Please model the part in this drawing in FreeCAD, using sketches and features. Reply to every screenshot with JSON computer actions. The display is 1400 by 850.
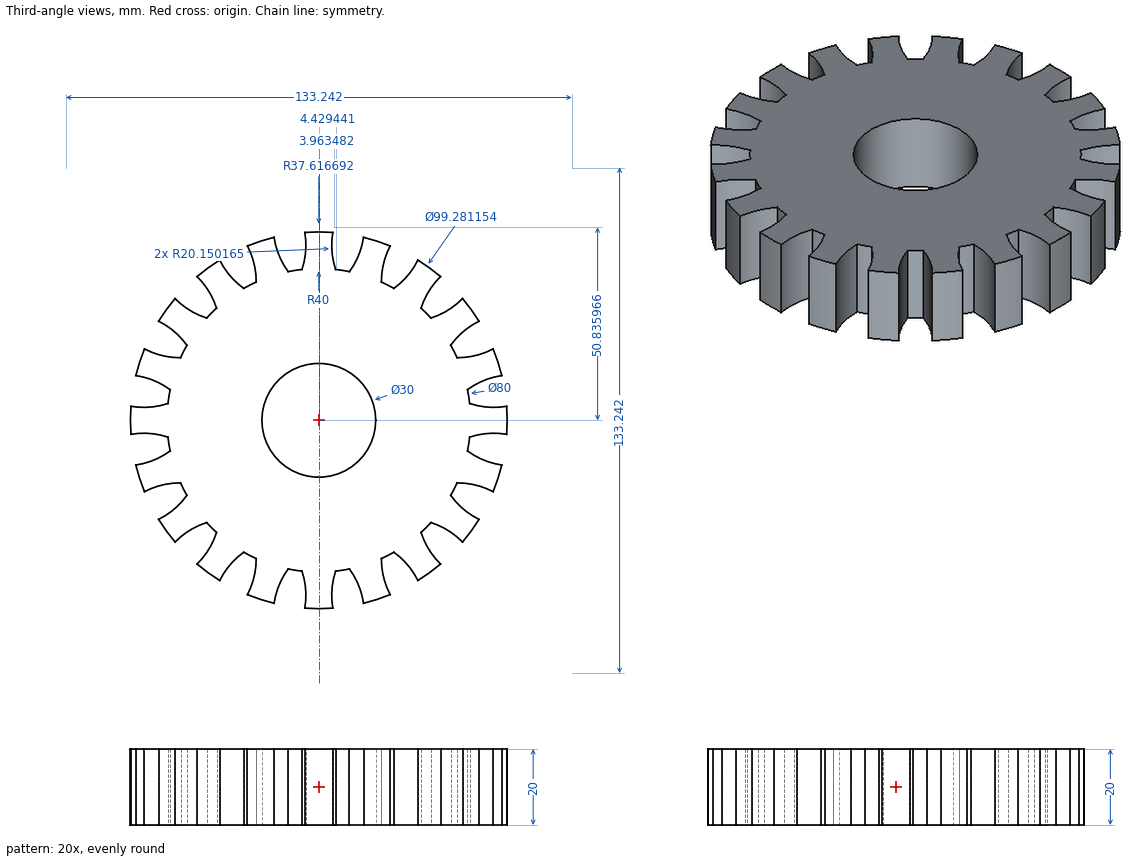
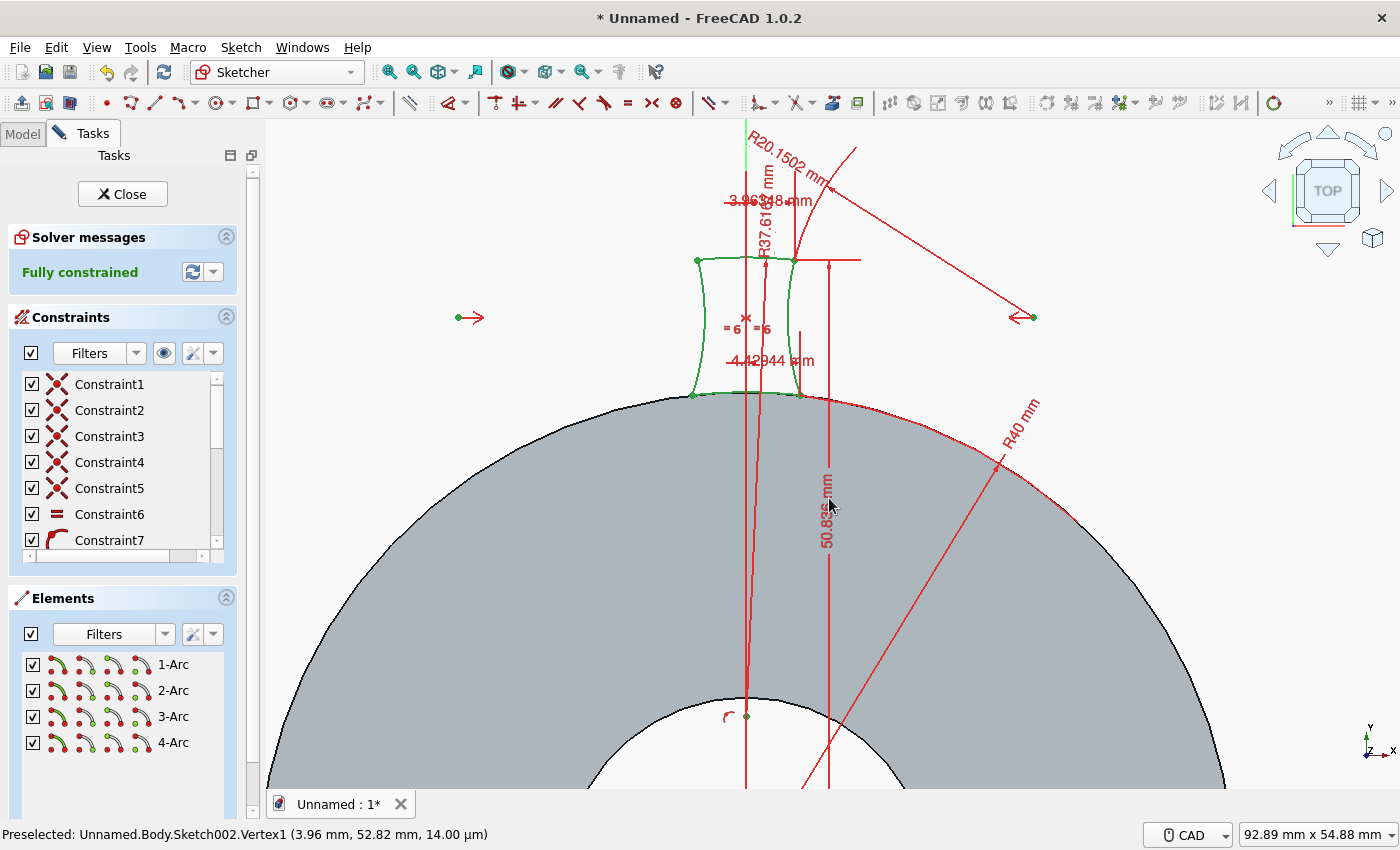
{"action": "left_click", "coordinate": [123, 194]}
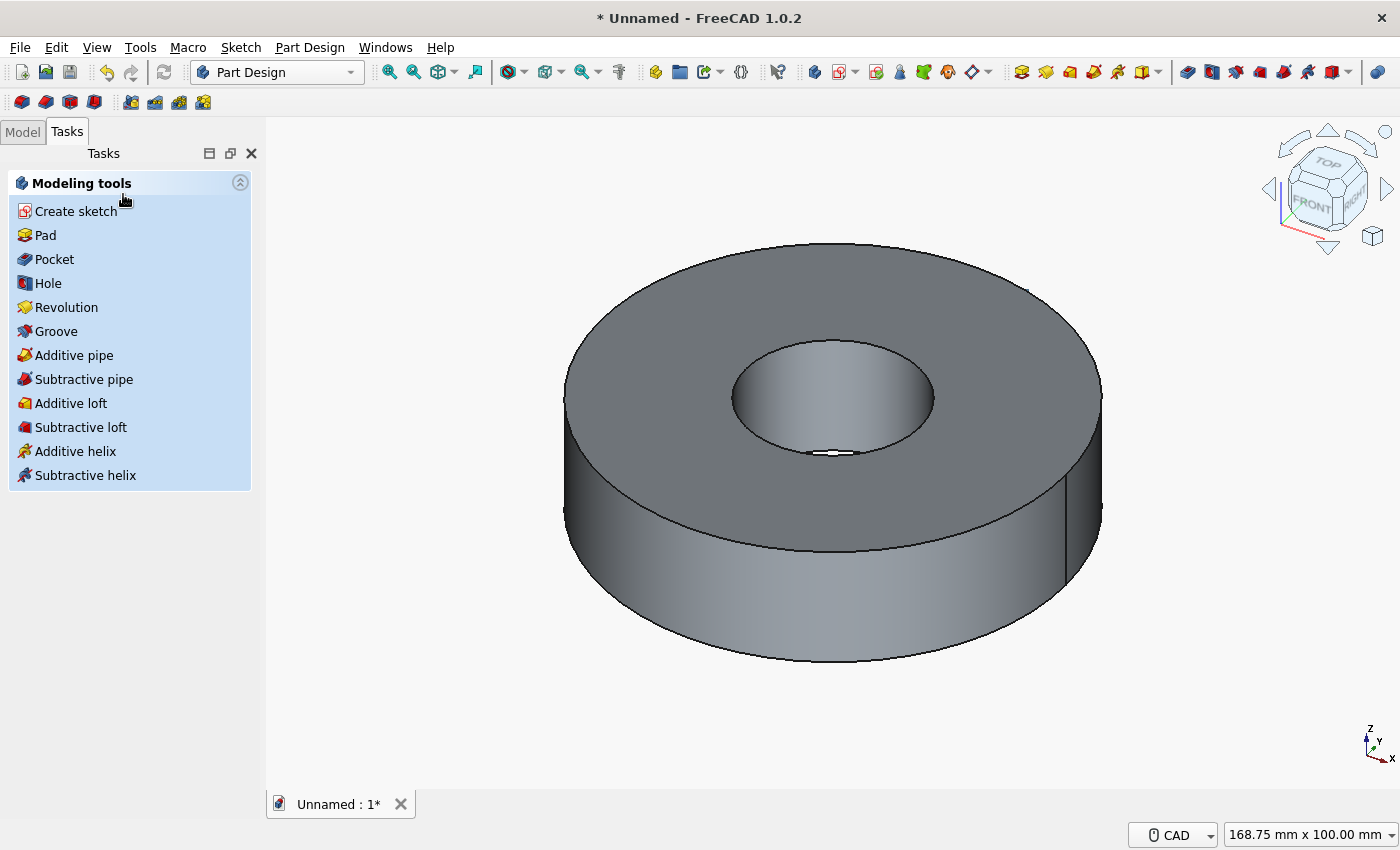
{"action": "left_click", "coordinate": [1022, 72]}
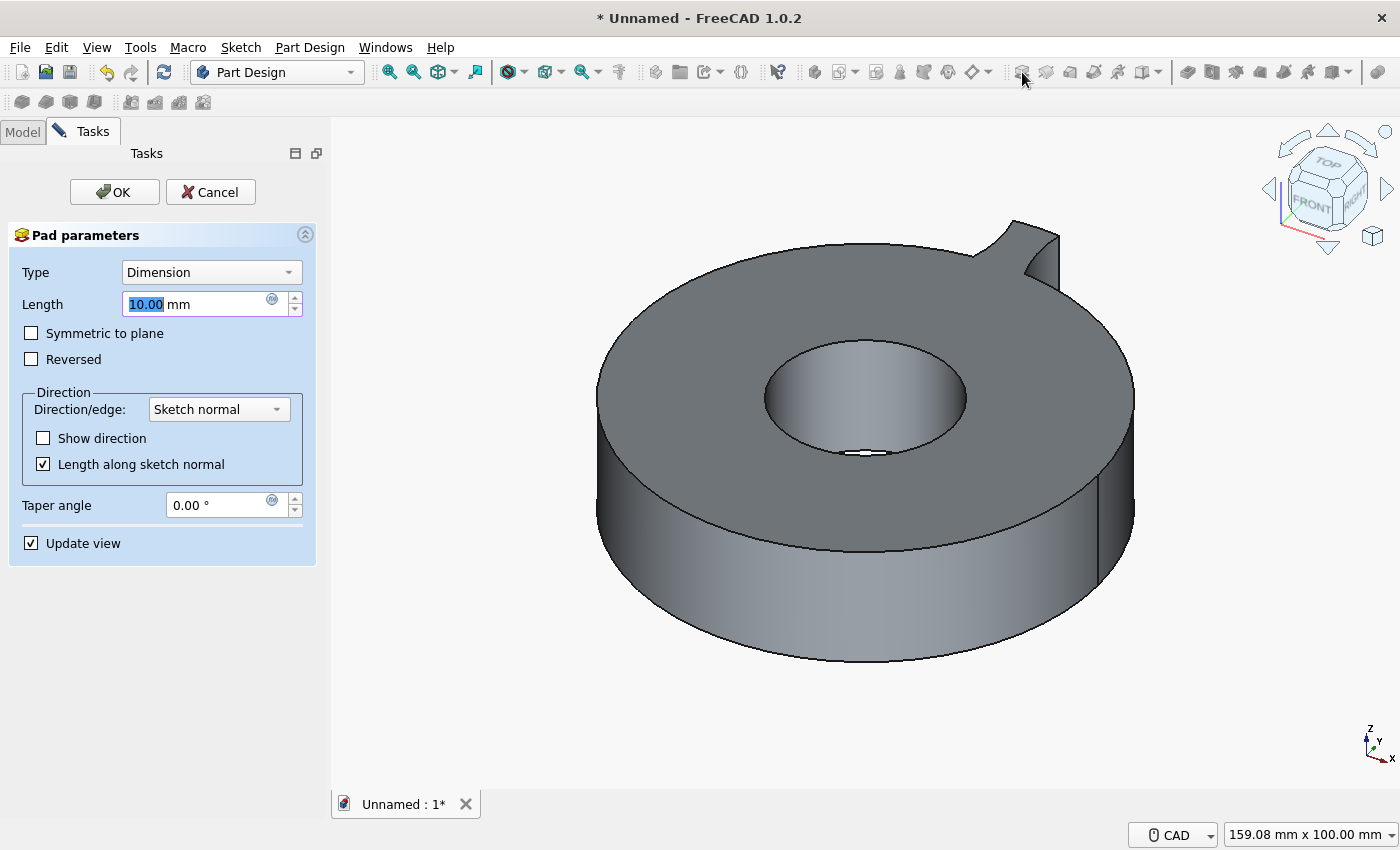
{"action": "type", "text": "20"}
{"action": "key", "text": "Tab"}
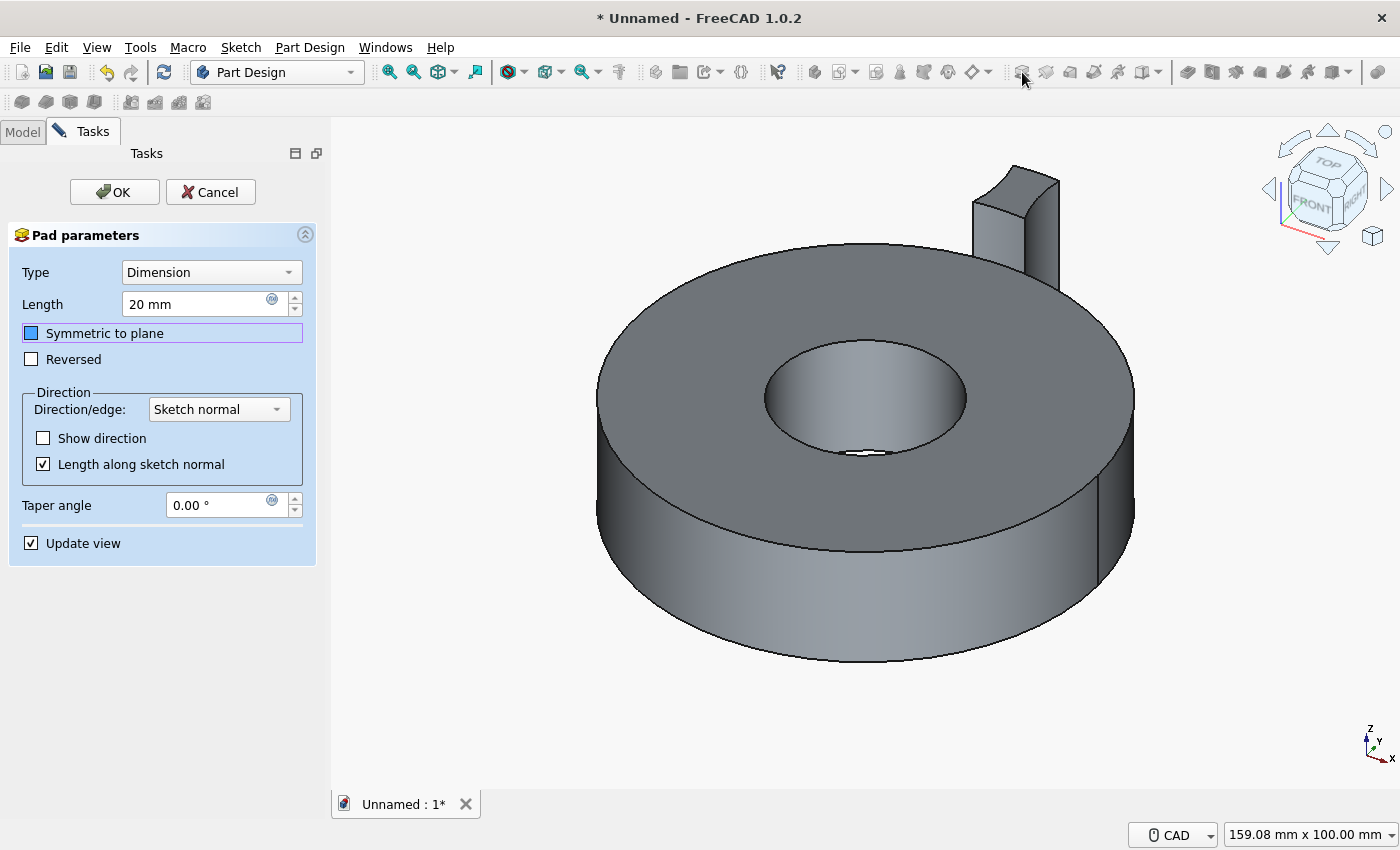
{"action": "left_click", "coordinate": [30, 333]}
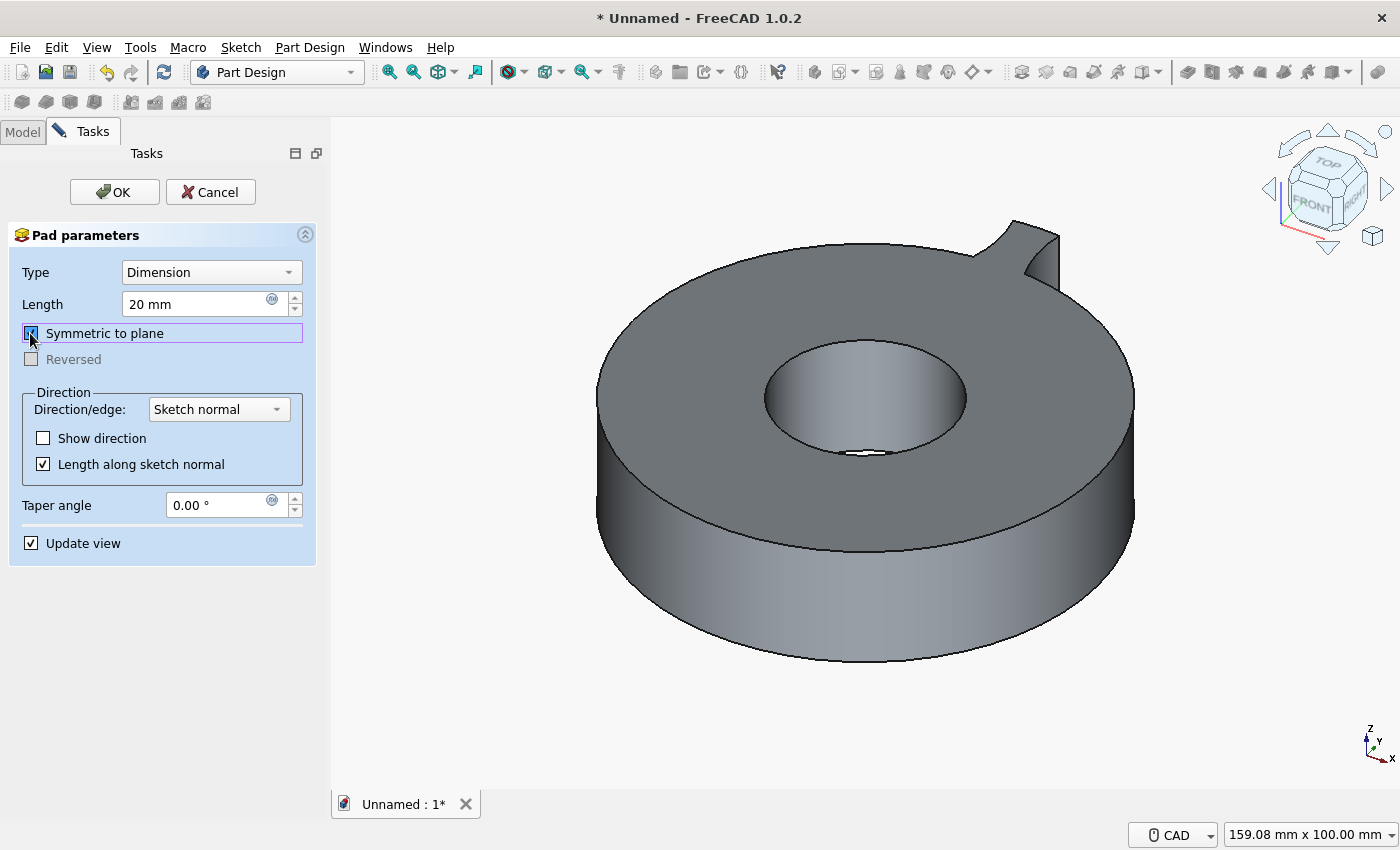
{"action": "left_click", "coordinate": [115, 192]}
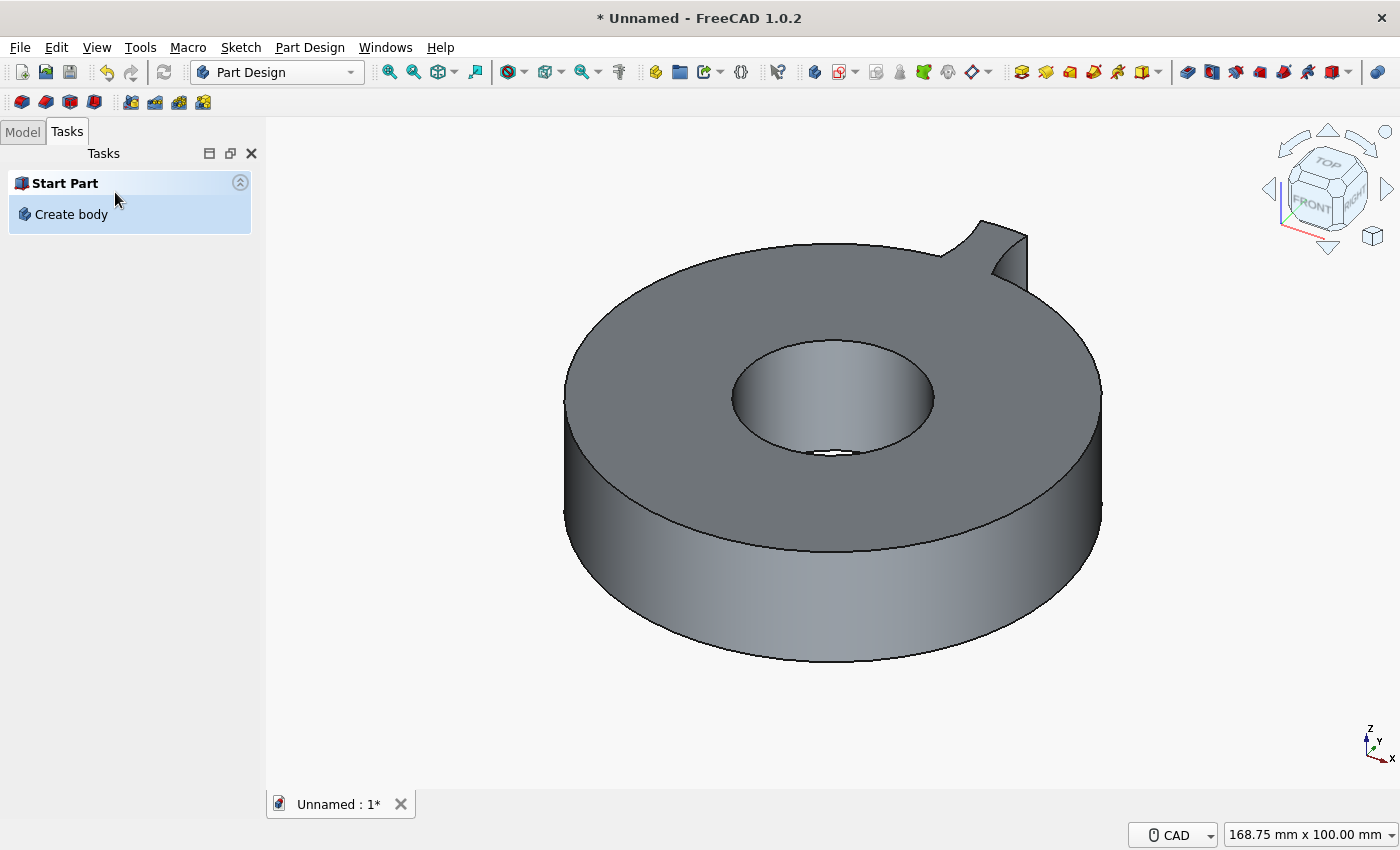
{"action": "left_click", "coordinate": [23, 131]}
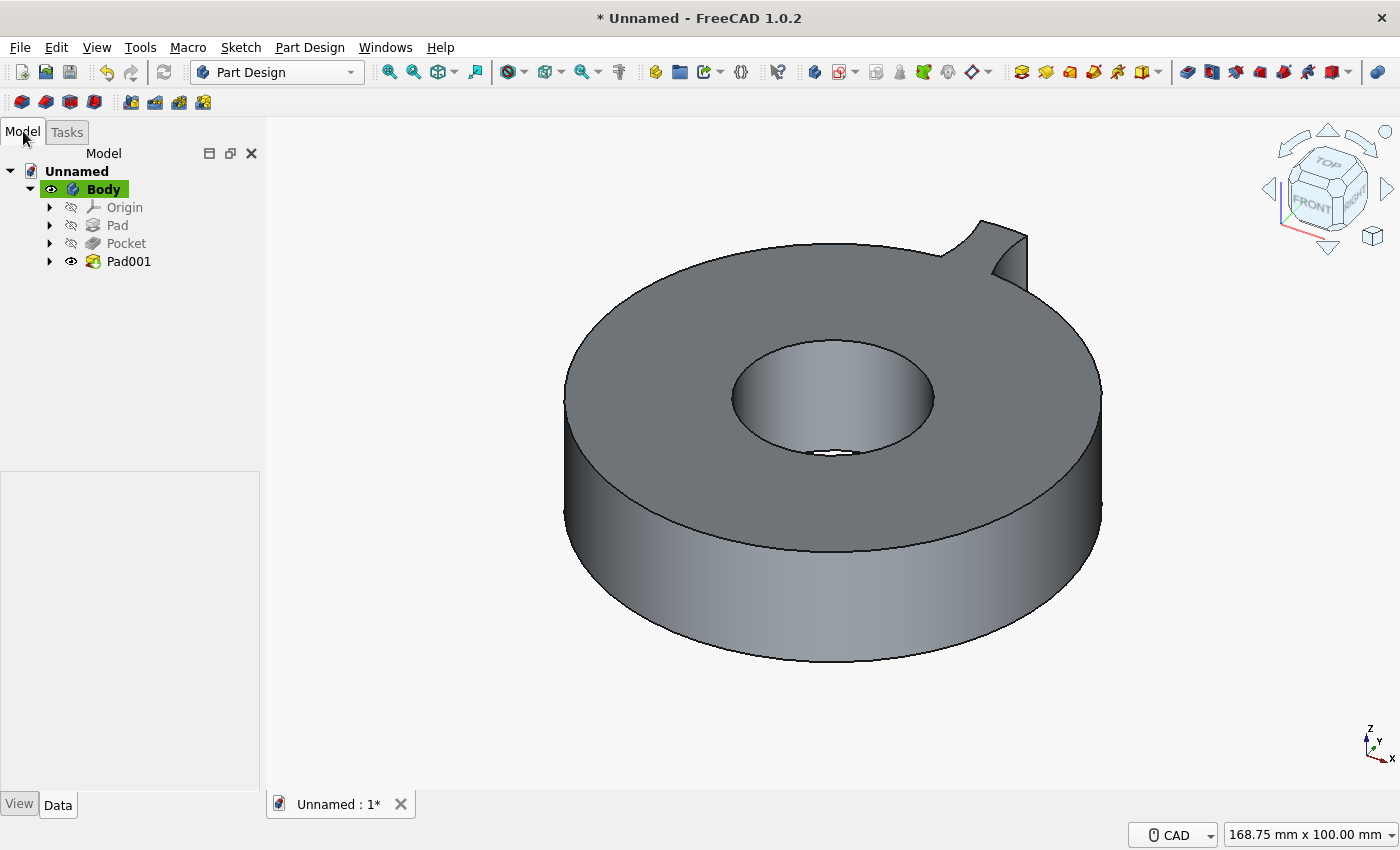
{"action": "left_click", "coordinate": [116, 261]}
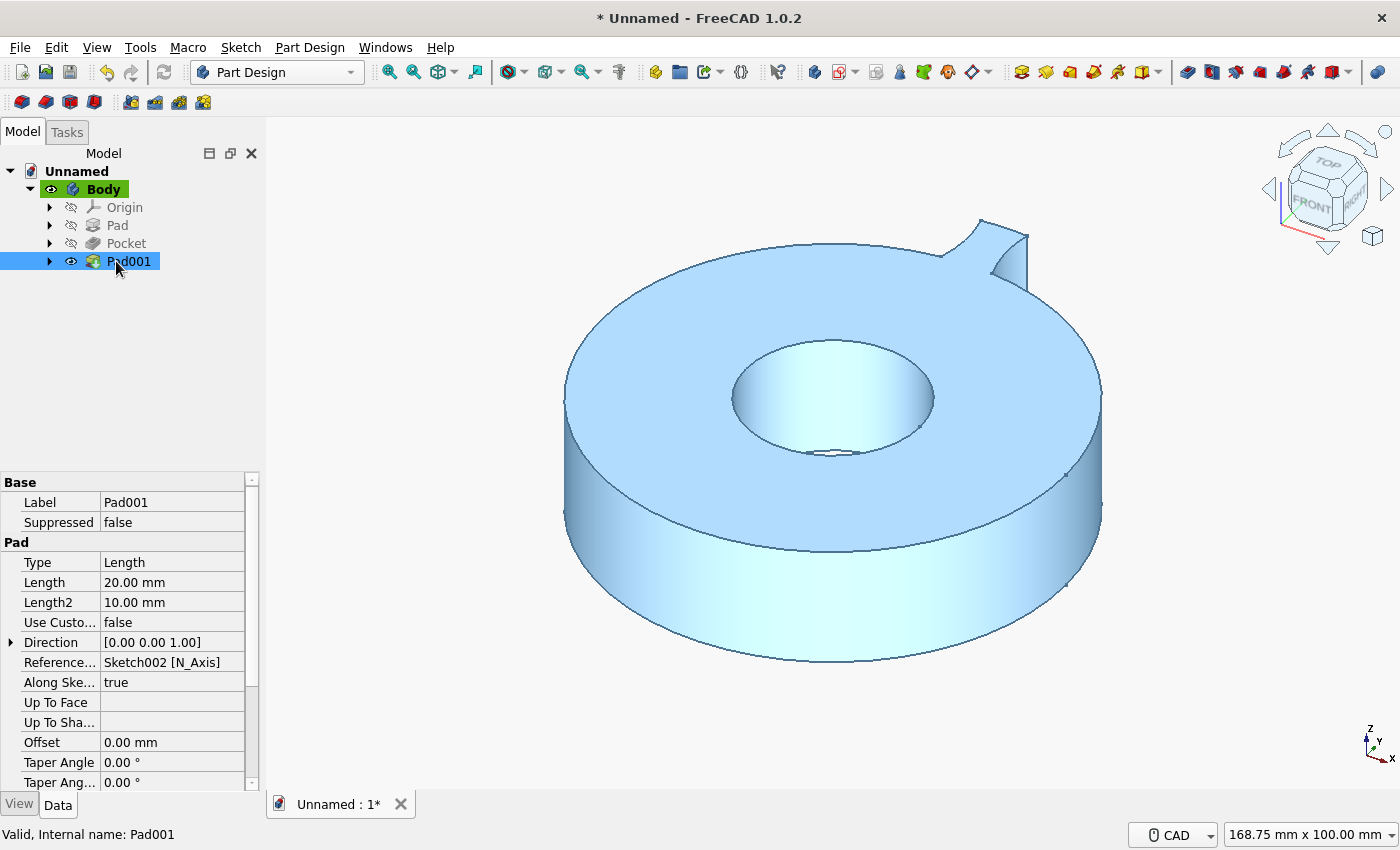
{"action": "left_click", "coordinate": [180, 102]}